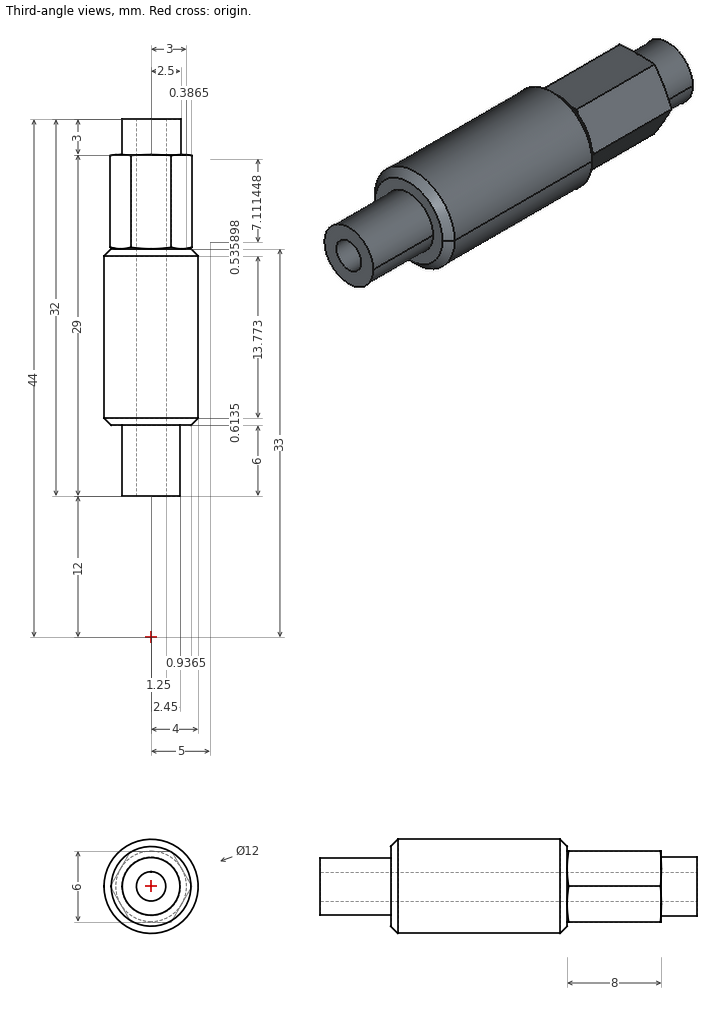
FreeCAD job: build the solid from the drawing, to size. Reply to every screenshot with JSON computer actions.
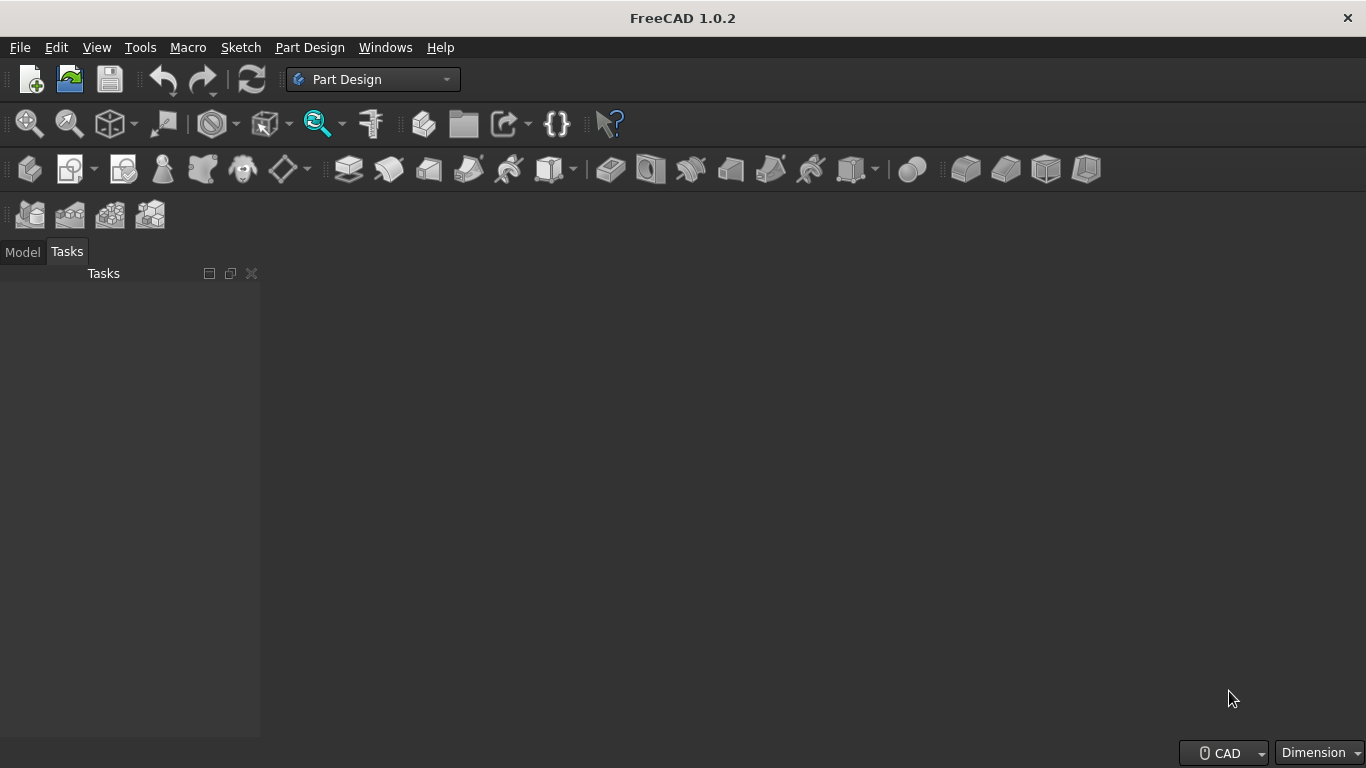
{"action": "left_click", "coordinate": [30, 80]}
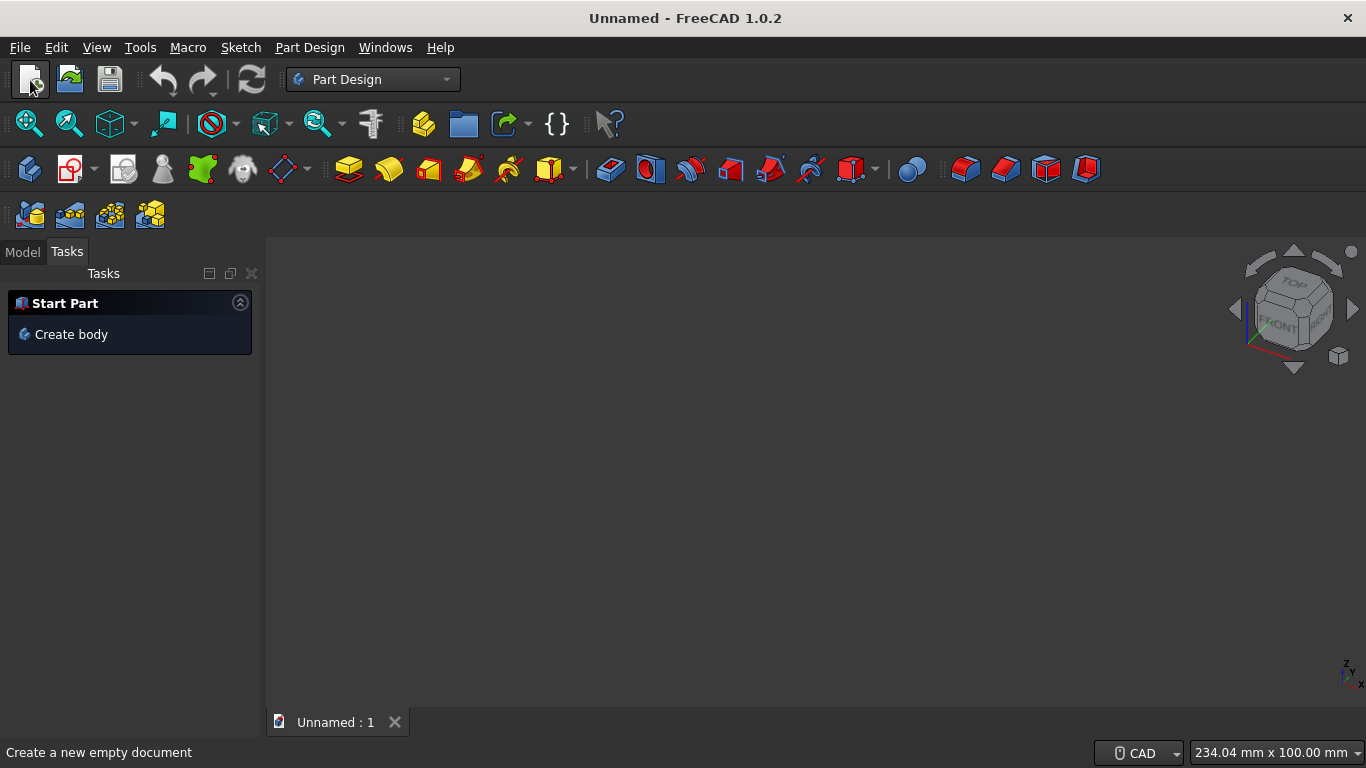
{"action": "left_click", "coordinate": [70, 170]}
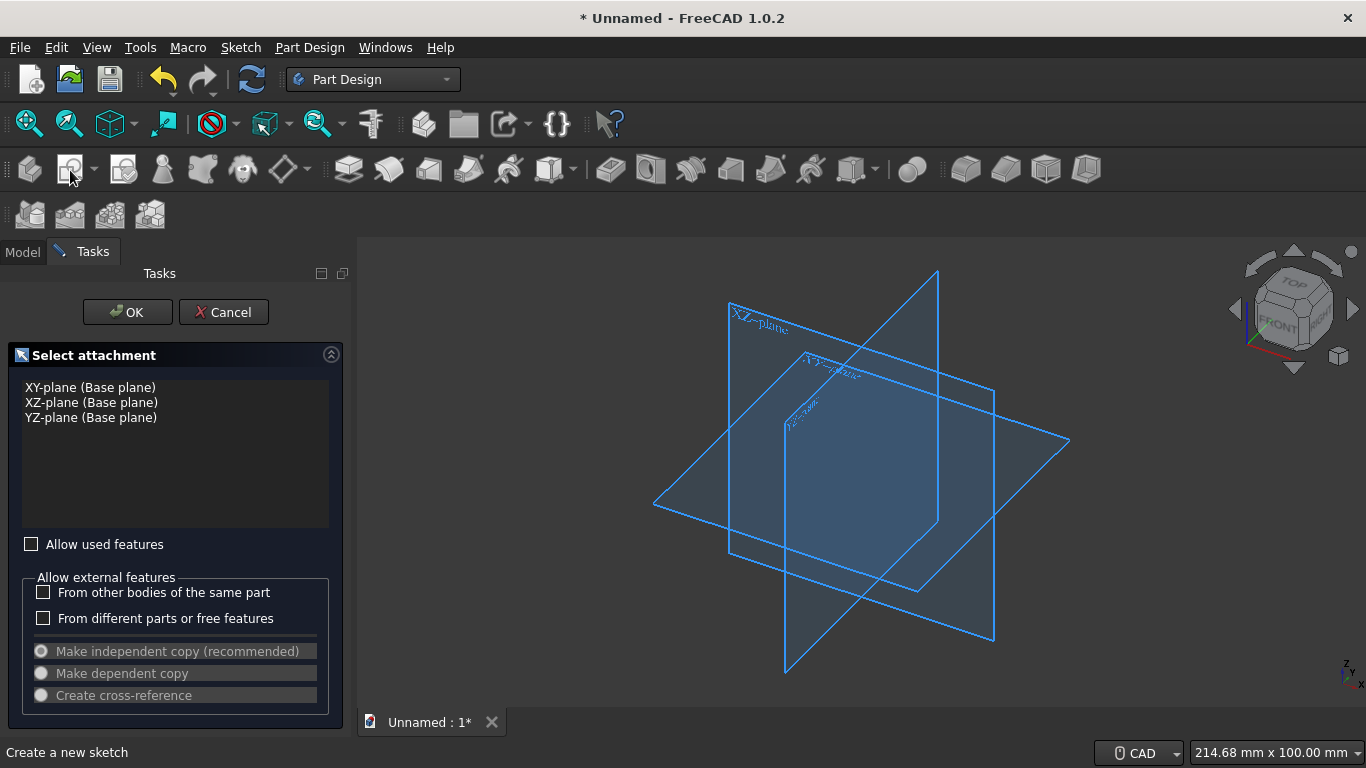
{"action": "left_click", "coordinate": [82, 388]}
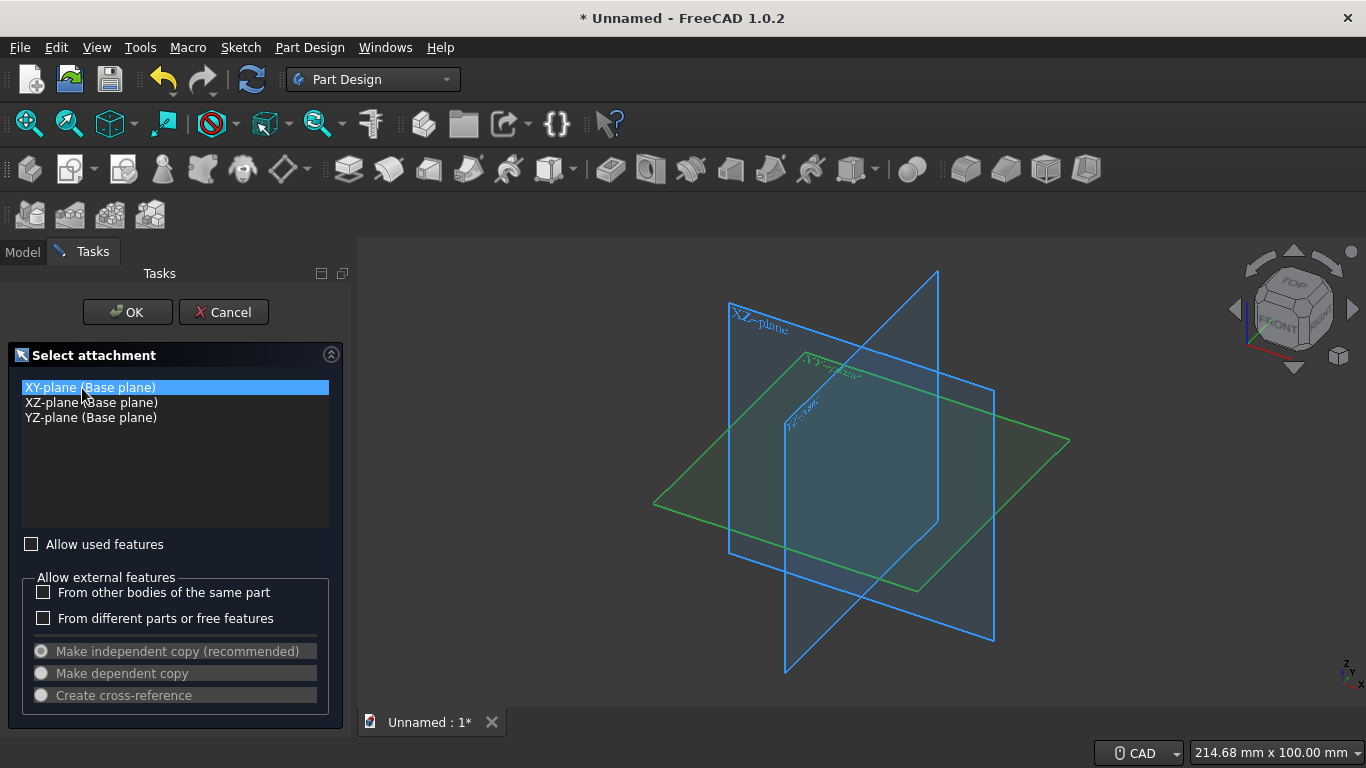
{"action": "left_click", "coordinate": [128, 312]}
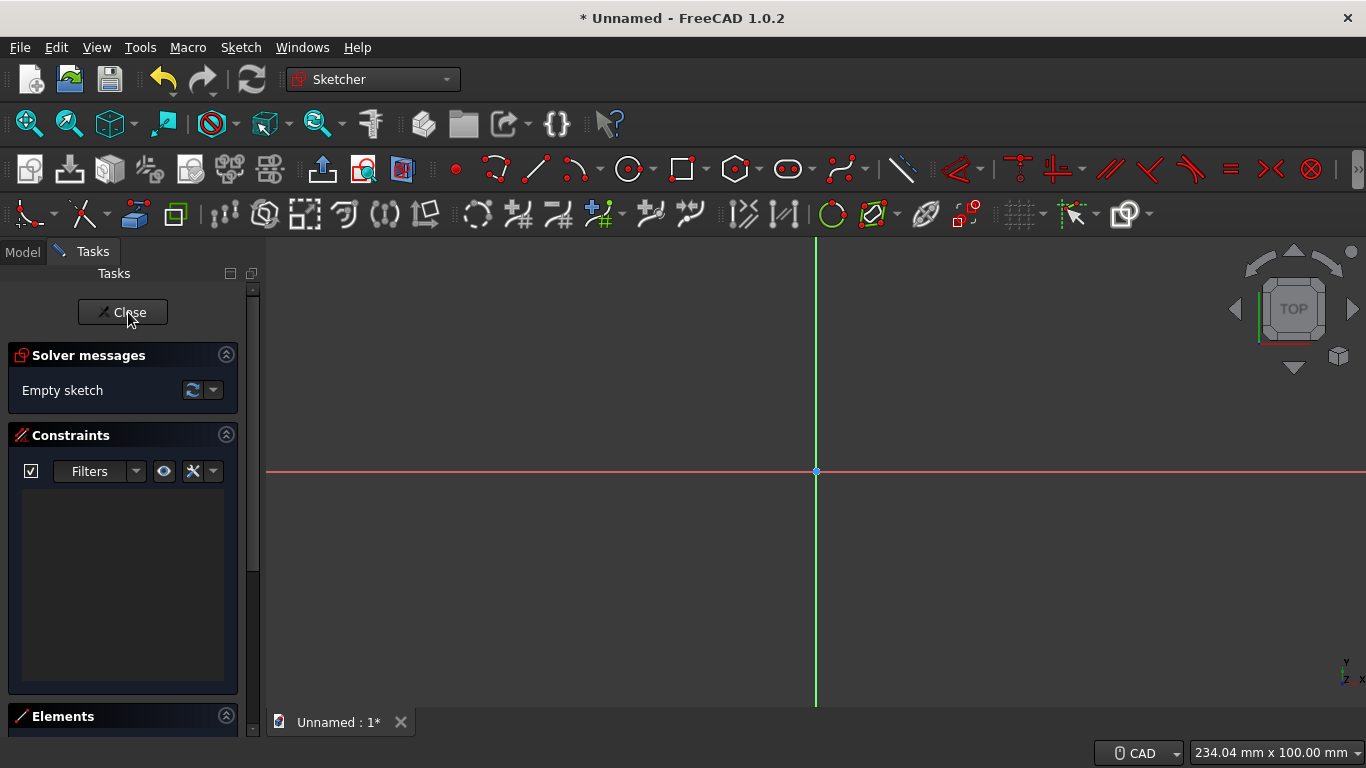
{"action": "scroll", "coordinate": [385, 679], "scroll_direction": "down", "scroll_amount": 1}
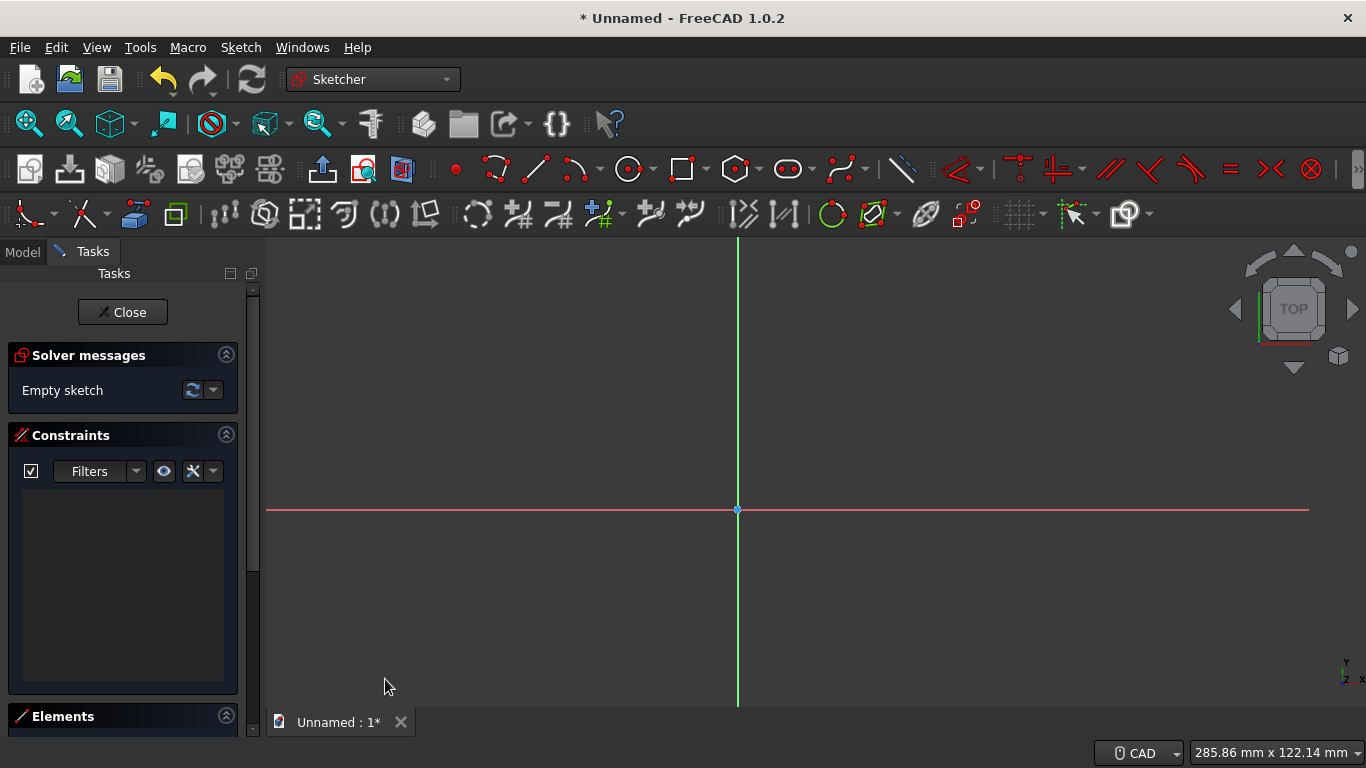
{"action": "scroll", "coordinate": [748, 381], "scroll_direction": "up", "scroll_amount": 3}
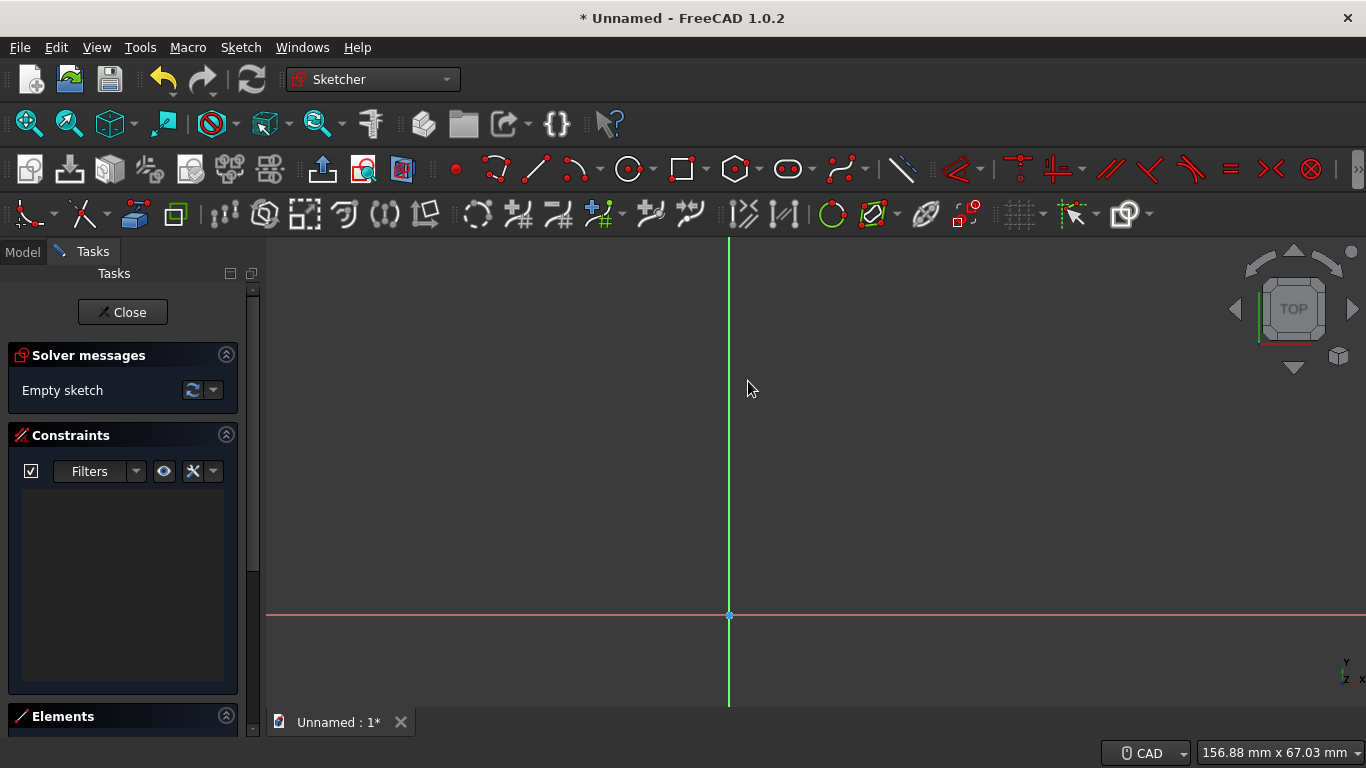
{"action": "left_click", "coordinate": [496, 170]}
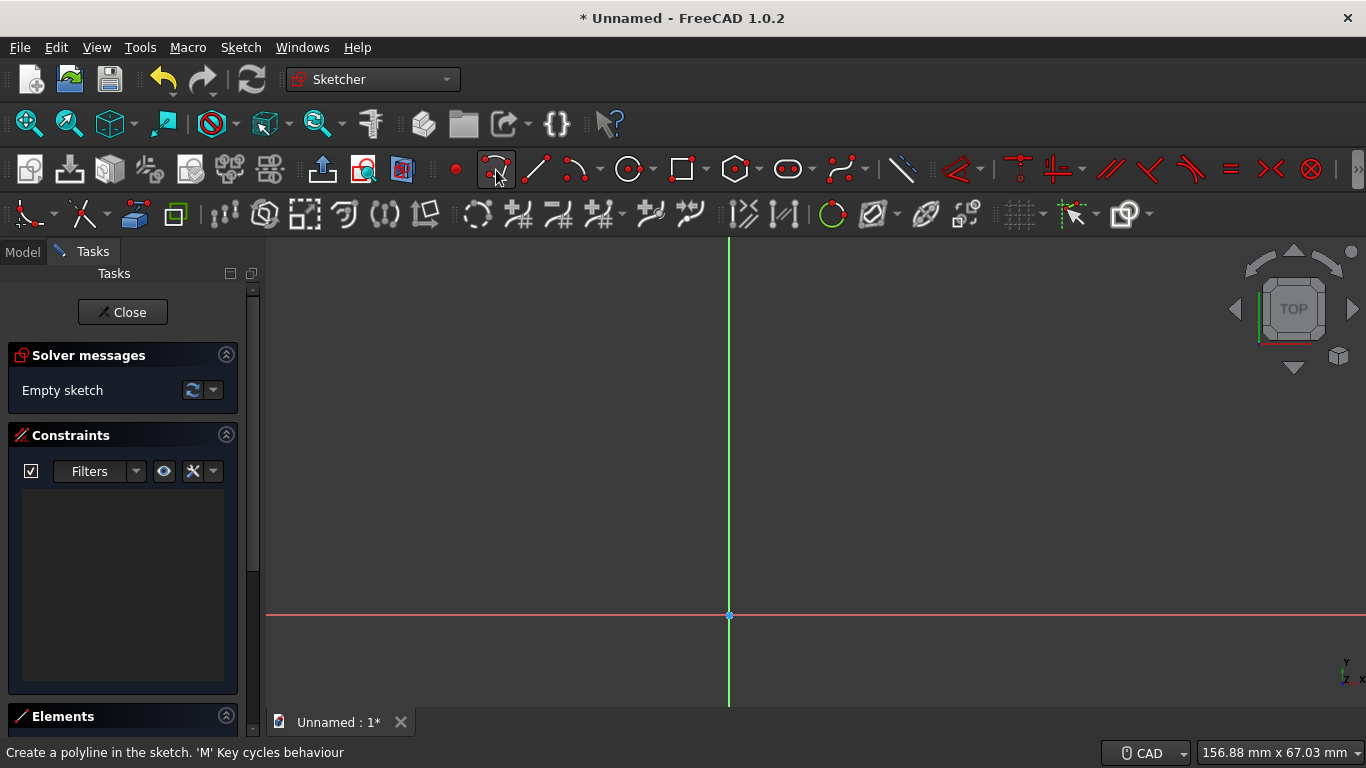
{"action": "left_click", "coordinate": [729, 531]}
{"action": "left_click", "coordinate": [746, 531]}
{"action": "left_click", "coordinate": [746, 489]}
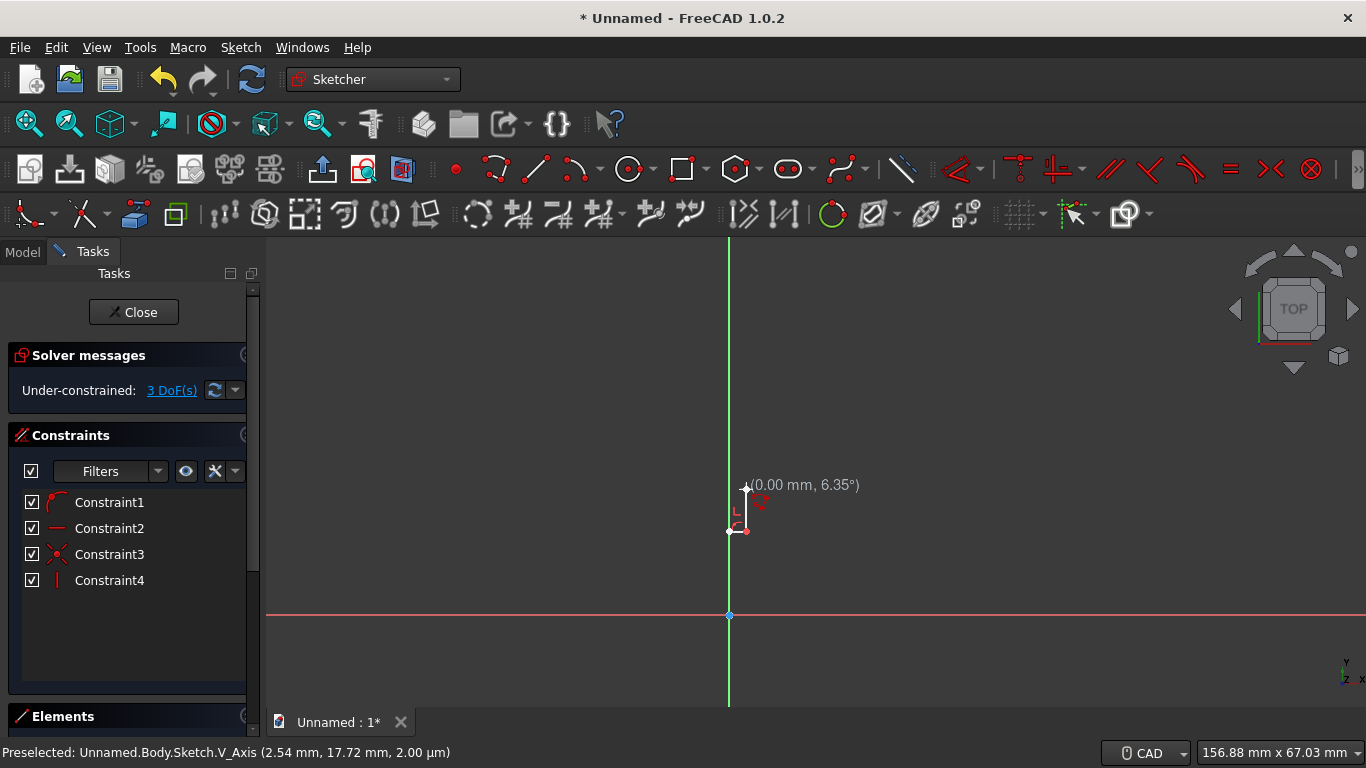
{"action": "scroll", "coordinate": [753, 489], "scroll_direction": "up", "scroll_amount": 5}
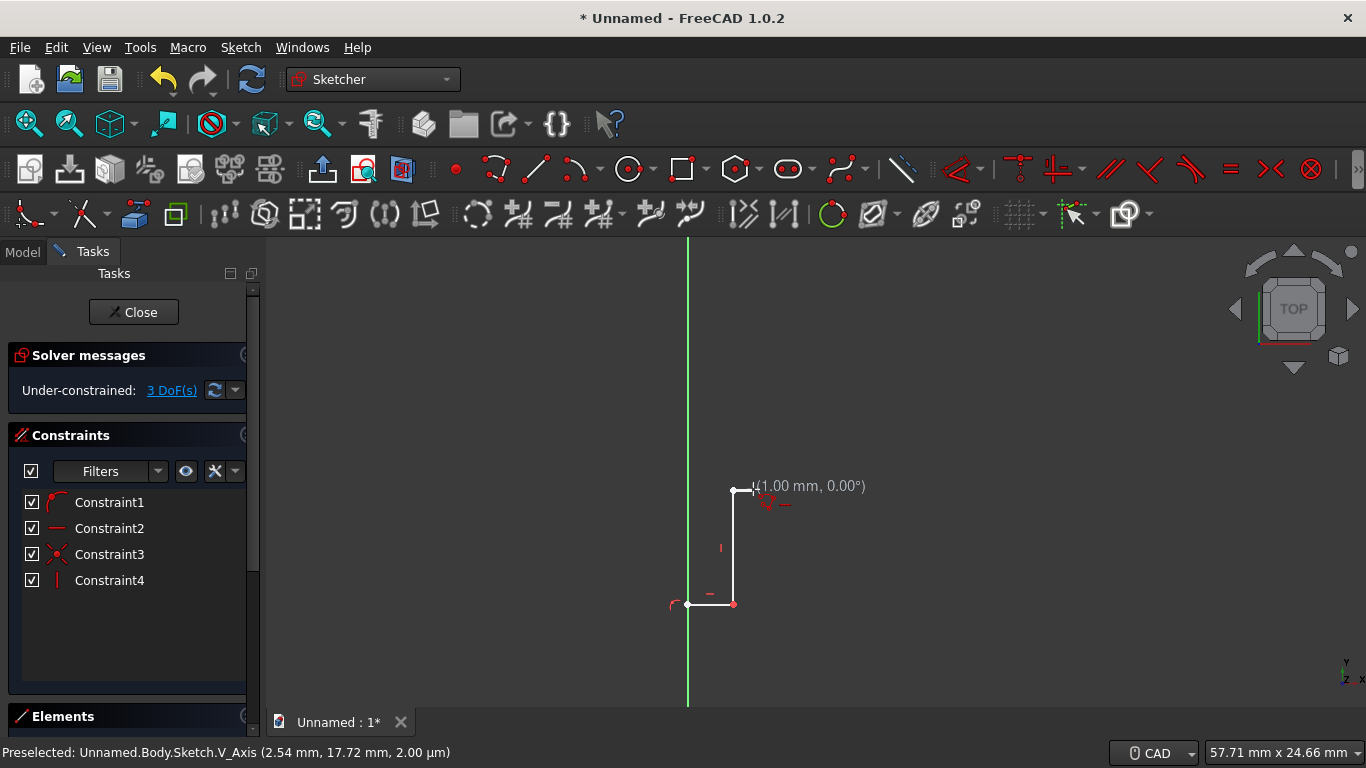
{"action": "left_click", "coordinate": [752, 488]}
{"action": "left_click", "coordinate": [764, 476]}